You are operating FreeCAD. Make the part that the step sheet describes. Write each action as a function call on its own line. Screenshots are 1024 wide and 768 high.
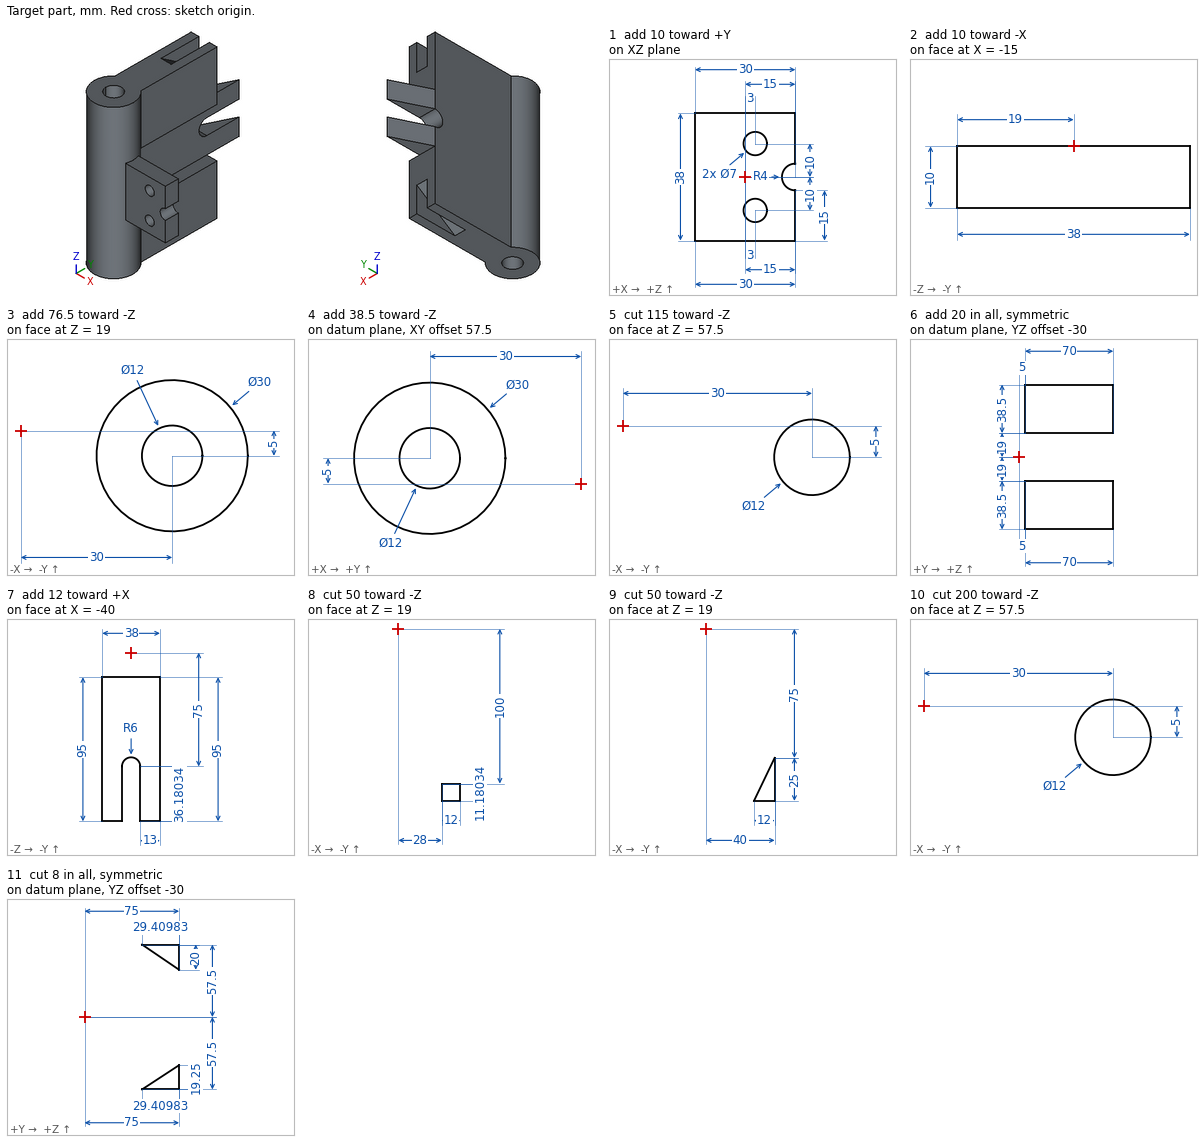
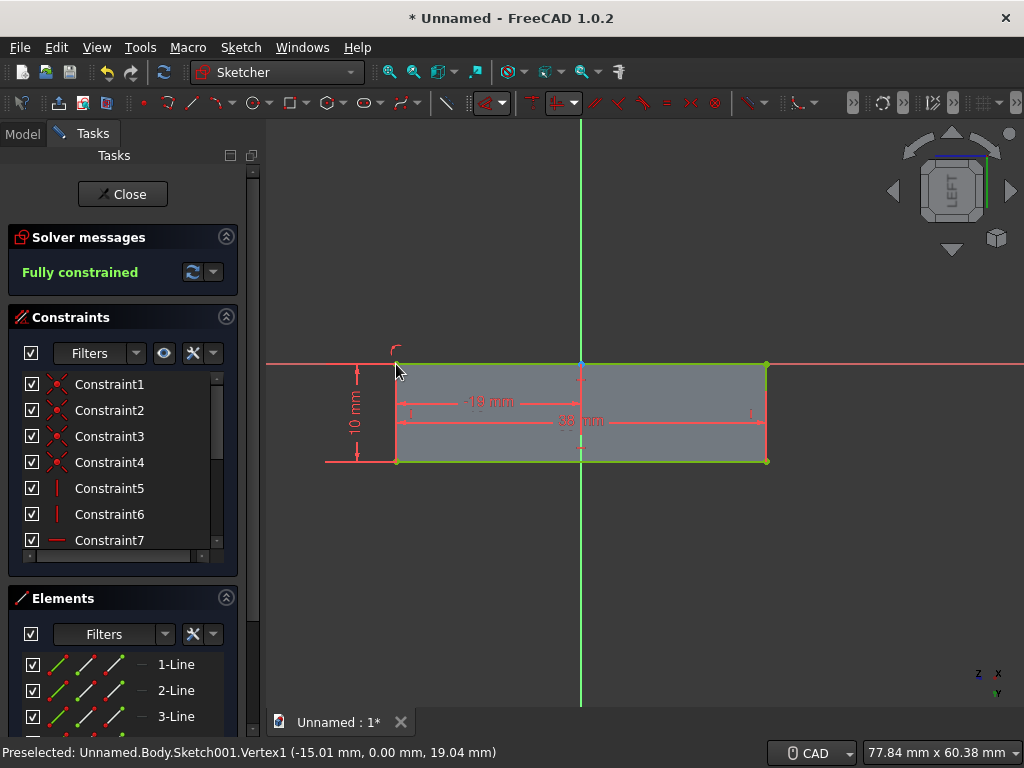
click(123, 194)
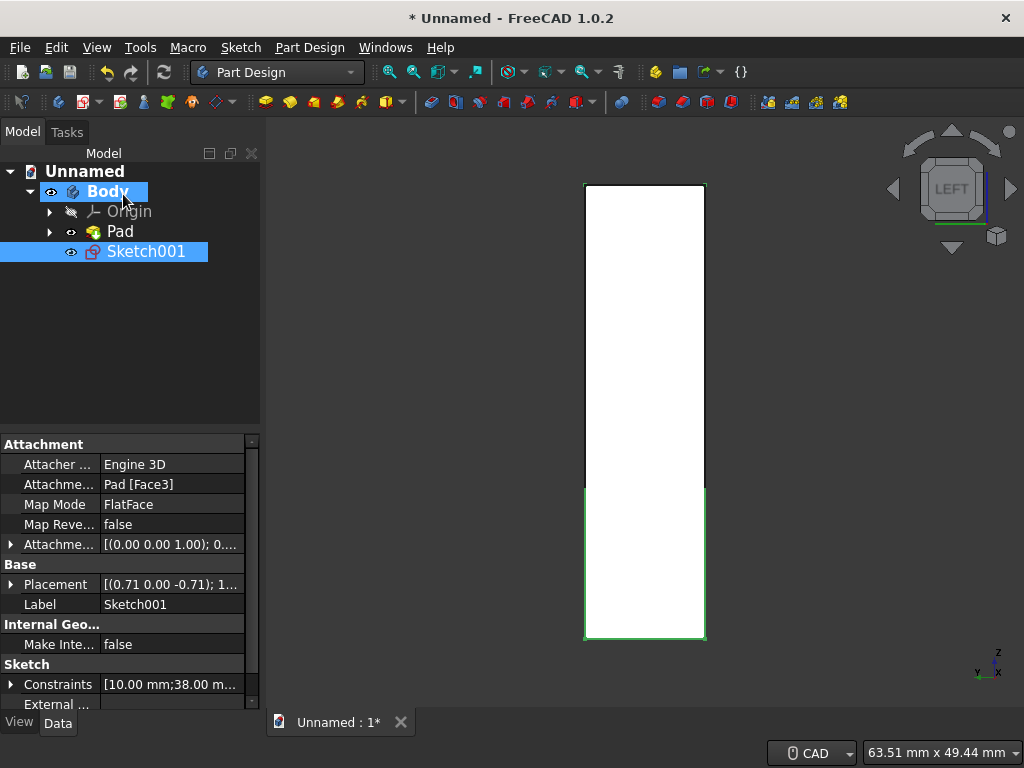
click(266, 102)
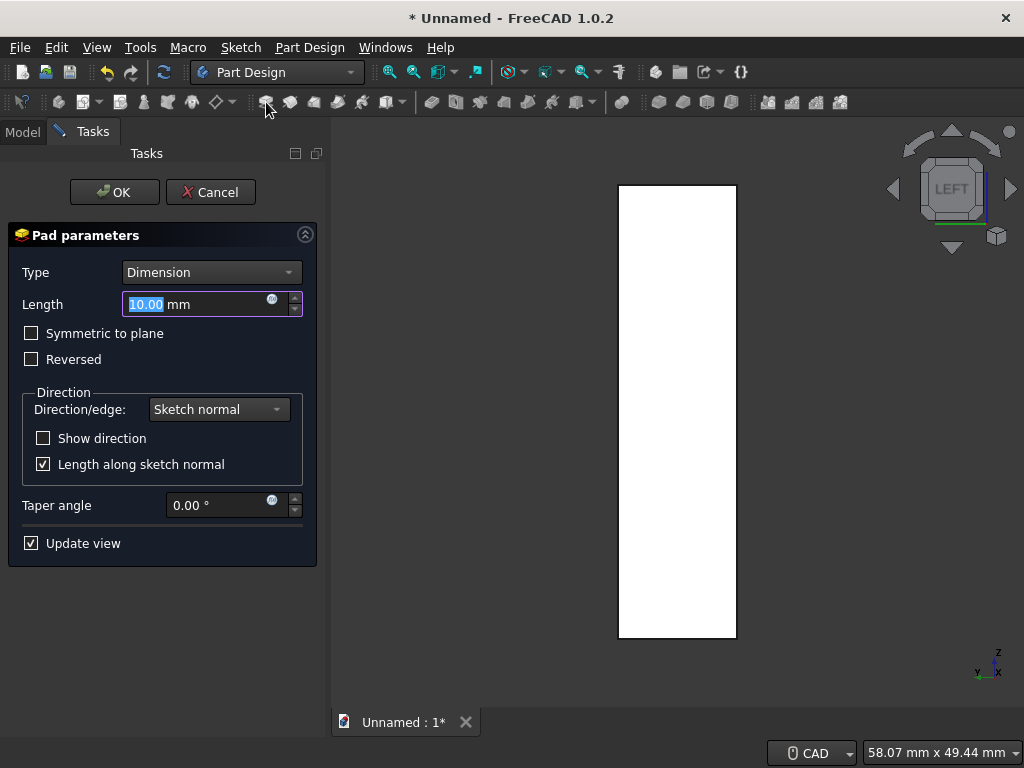
text(10)
key(Tab)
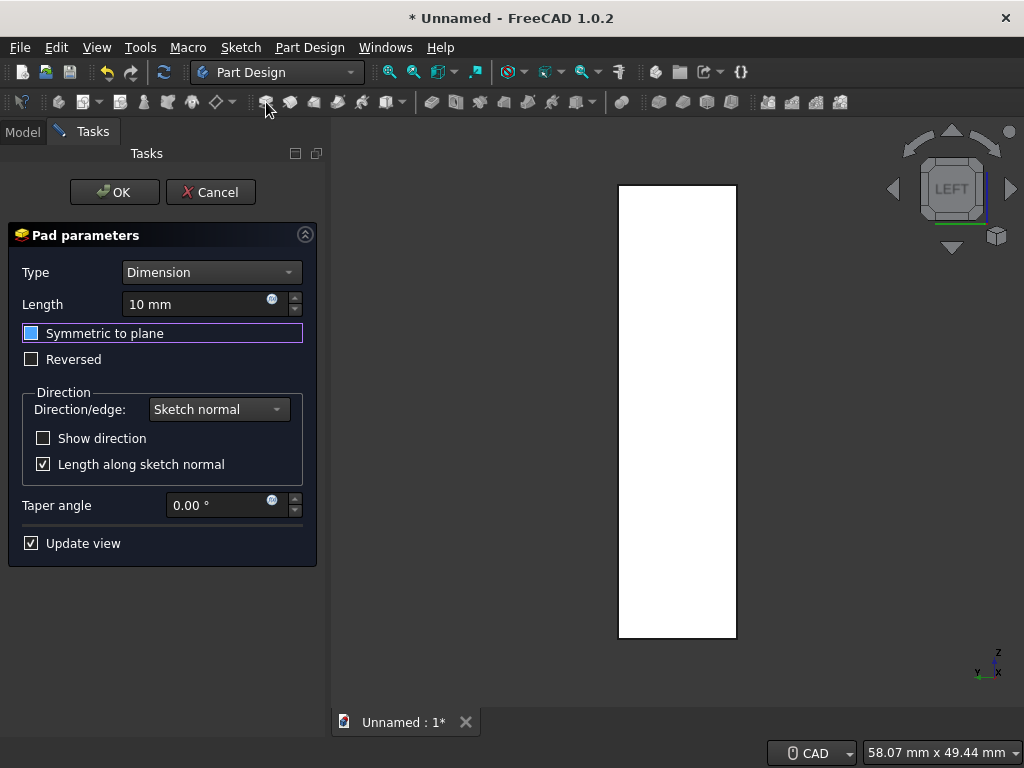
click(115, 192)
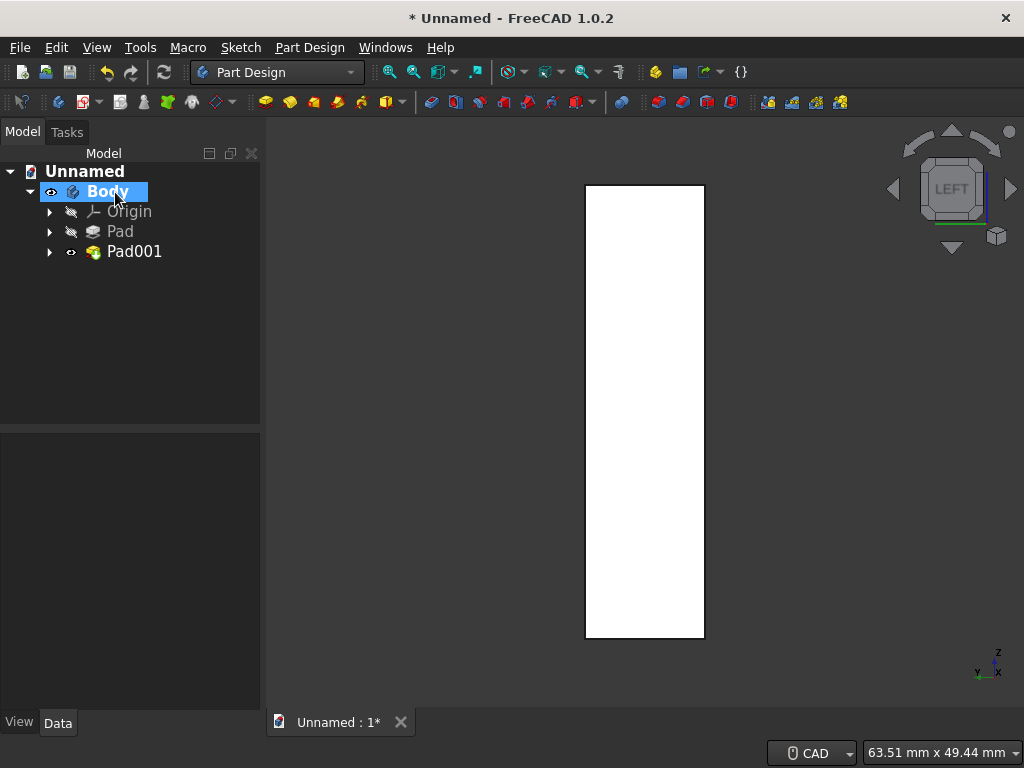
key(0)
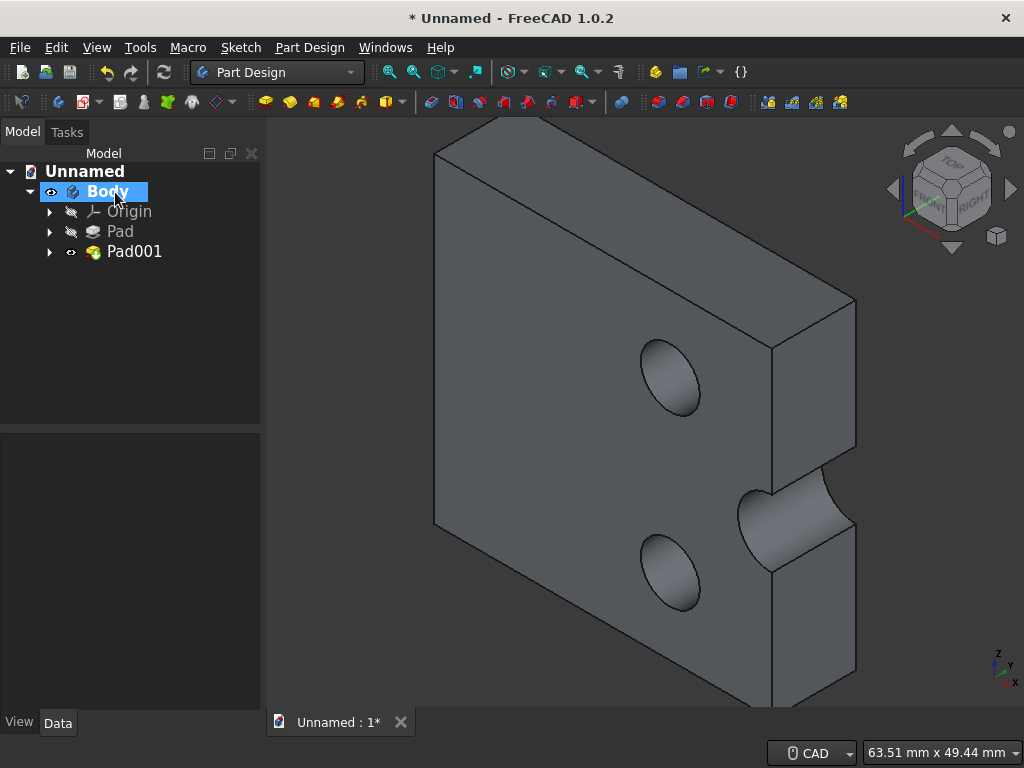
click(390, 72)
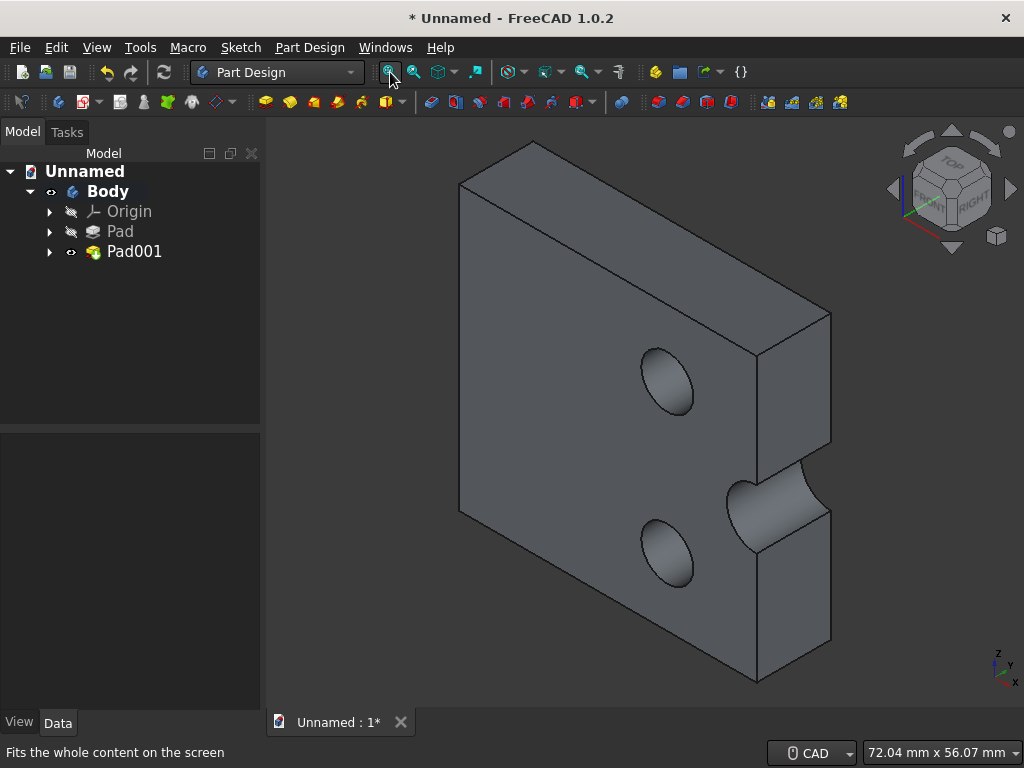
click(730, 297)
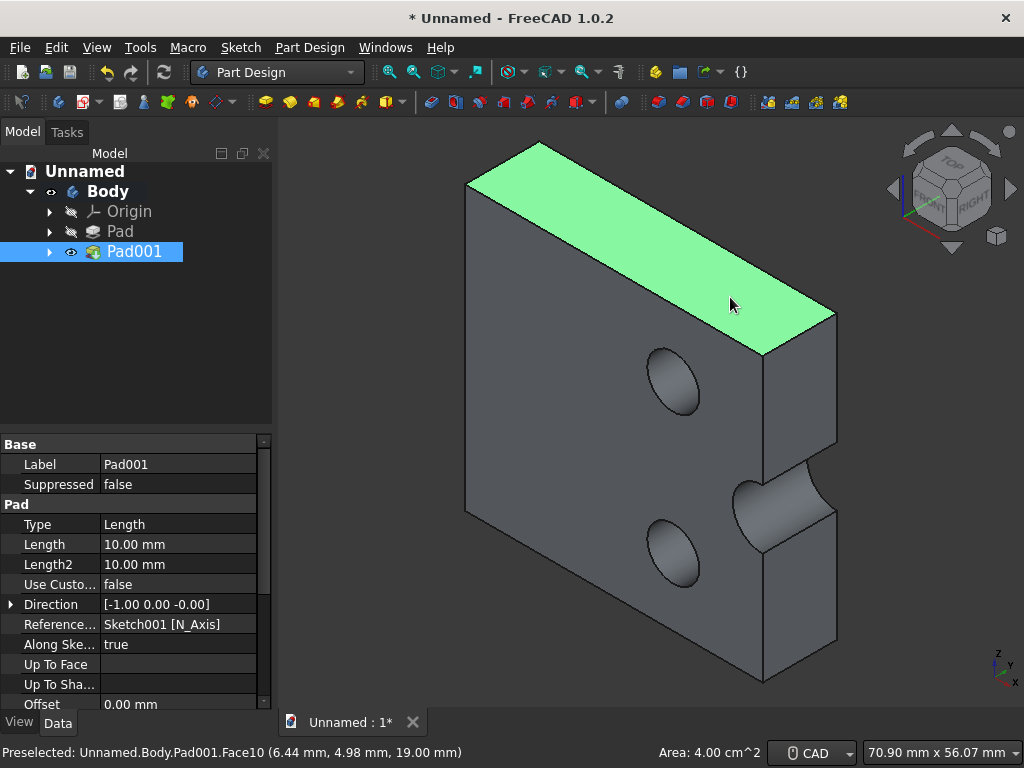
click(84, 102)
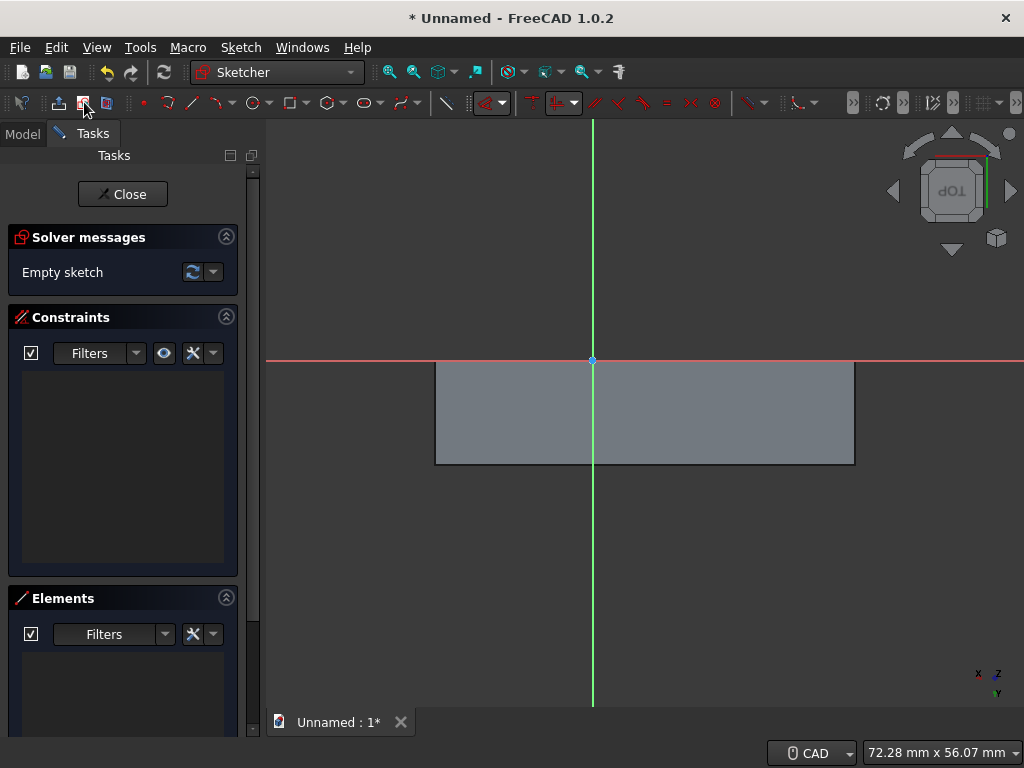
scroll(294, 413, down, 2)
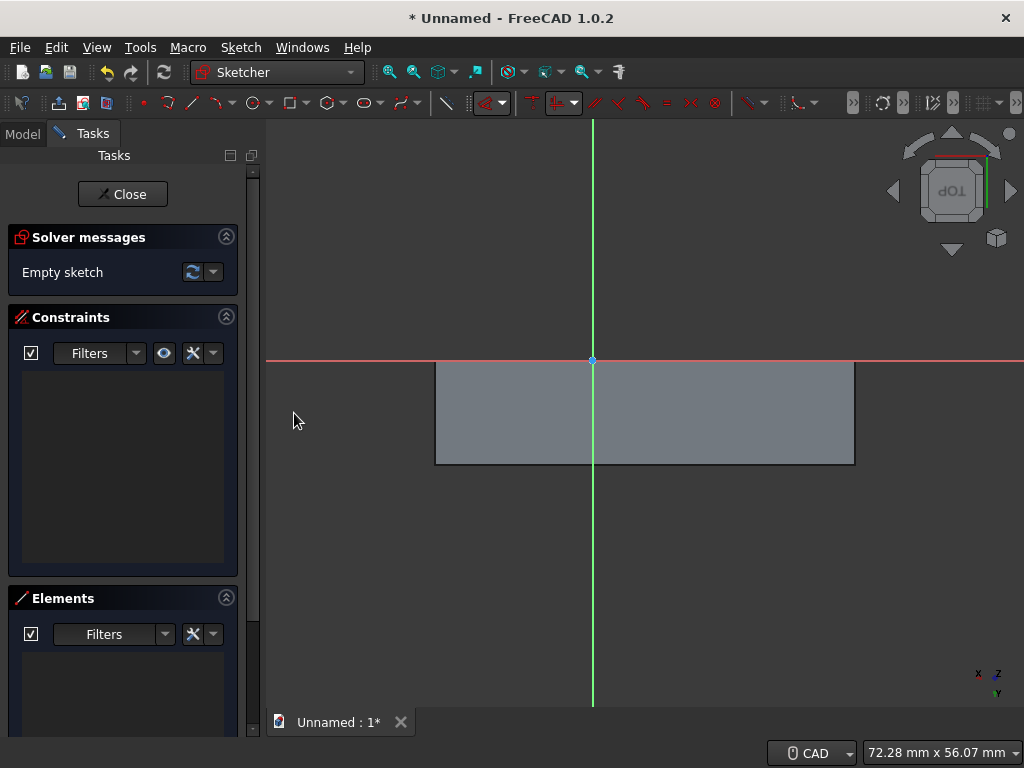
key(g)
key(c)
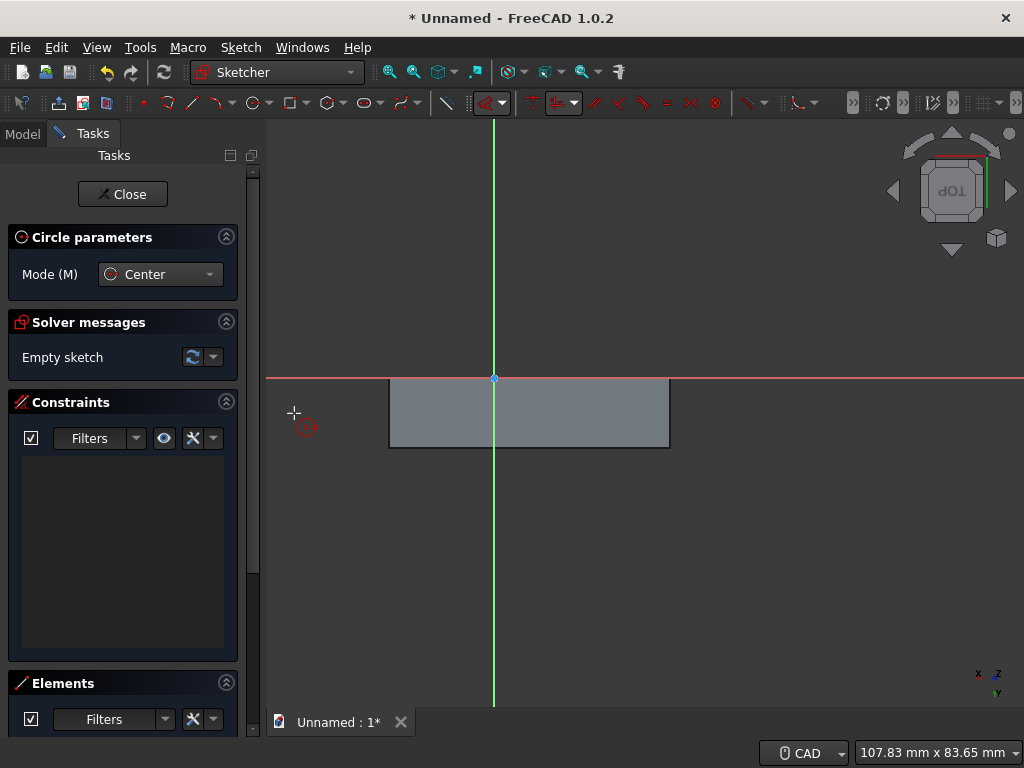
click(705, 413)
click(780, 339)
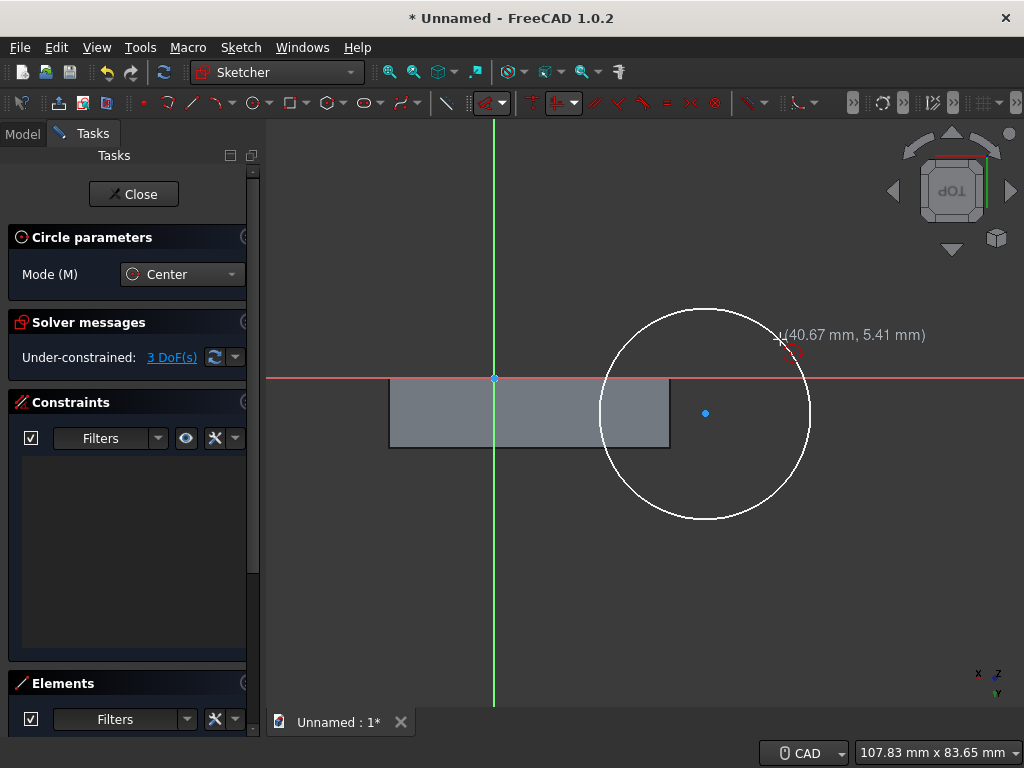
click(705, 414)
click(735, 443)
key(Escape)